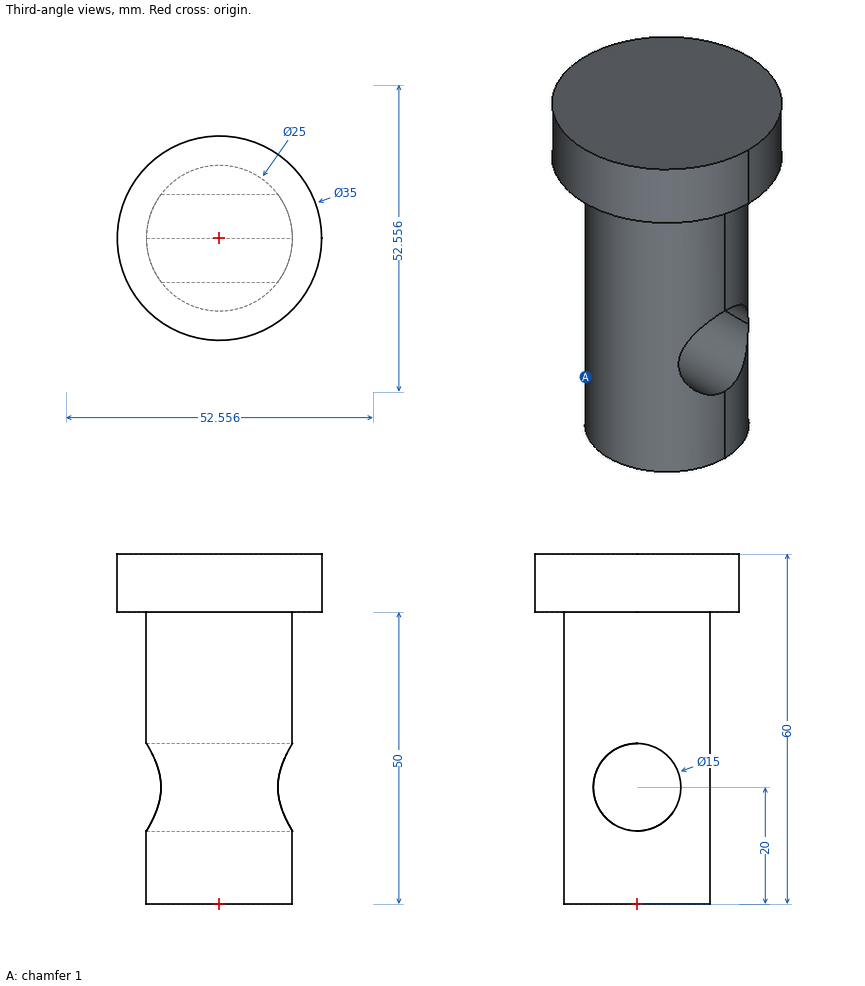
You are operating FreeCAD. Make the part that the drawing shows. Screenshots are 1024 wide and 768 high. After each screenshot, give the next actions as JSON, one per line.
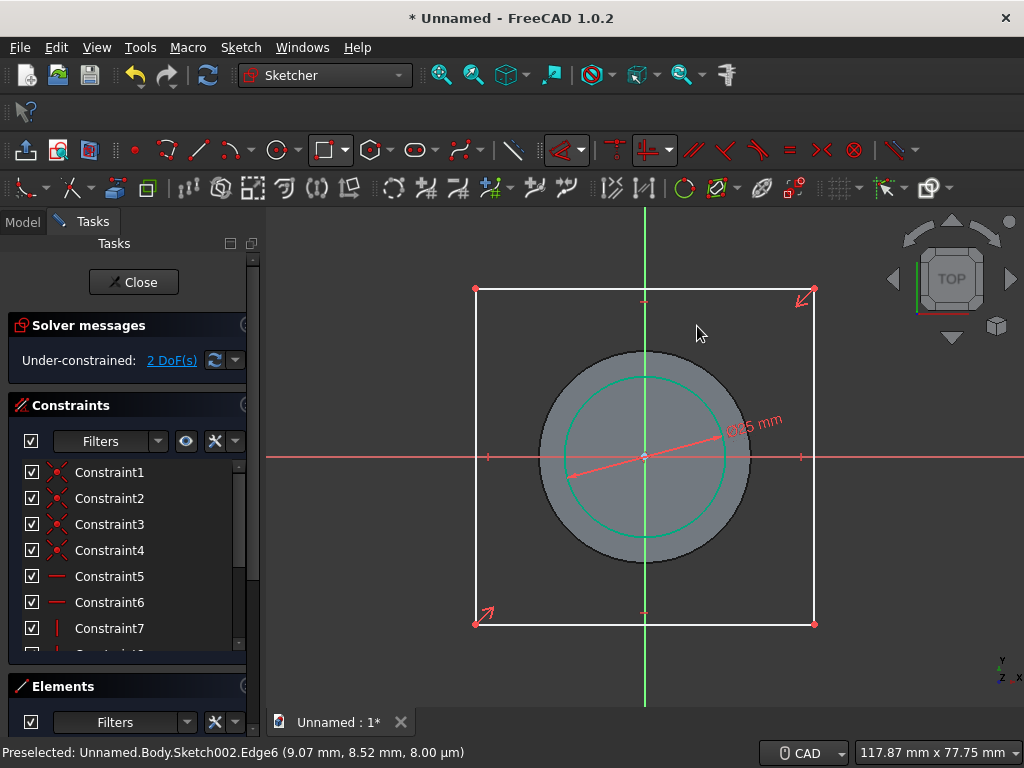
{"action": "left_click", "coordinate": [577, 625]}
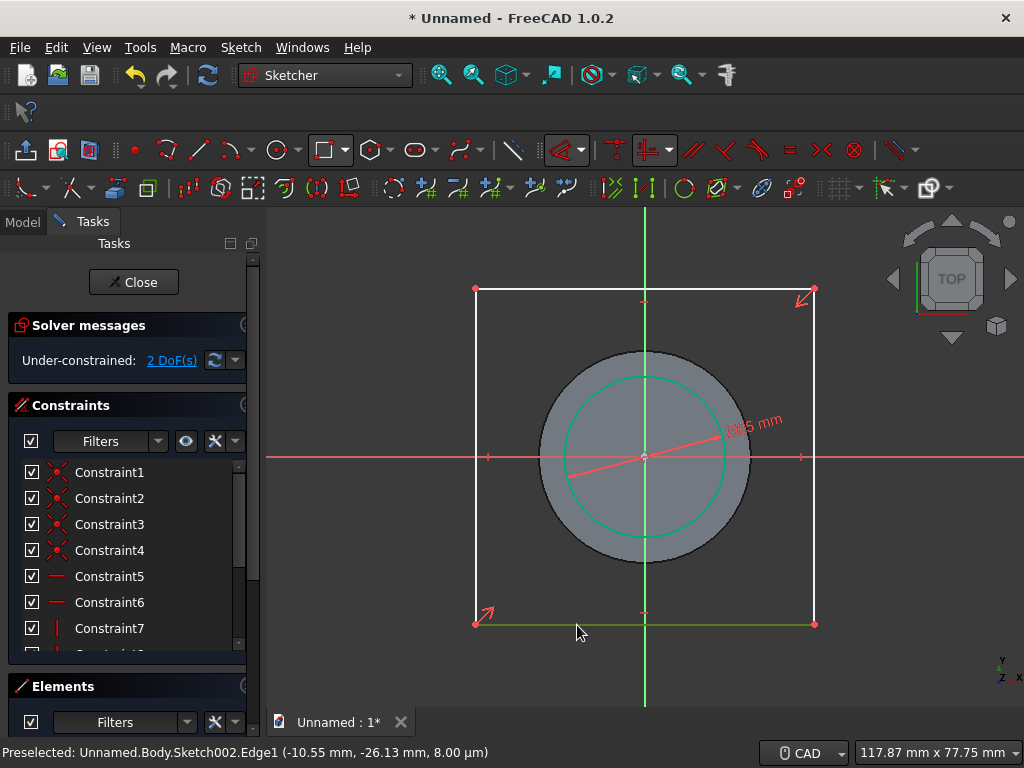
{"action": "left_click", "coordinate": [584, 150]}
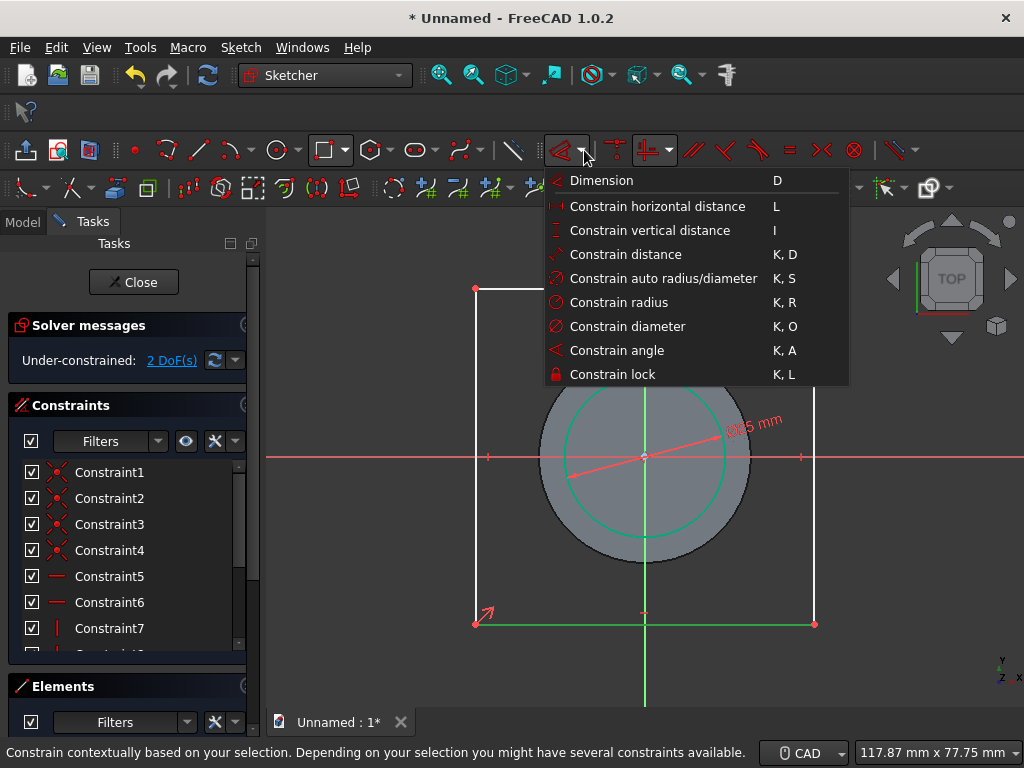
{"action": "left_click", "coordinate": [697, 206]}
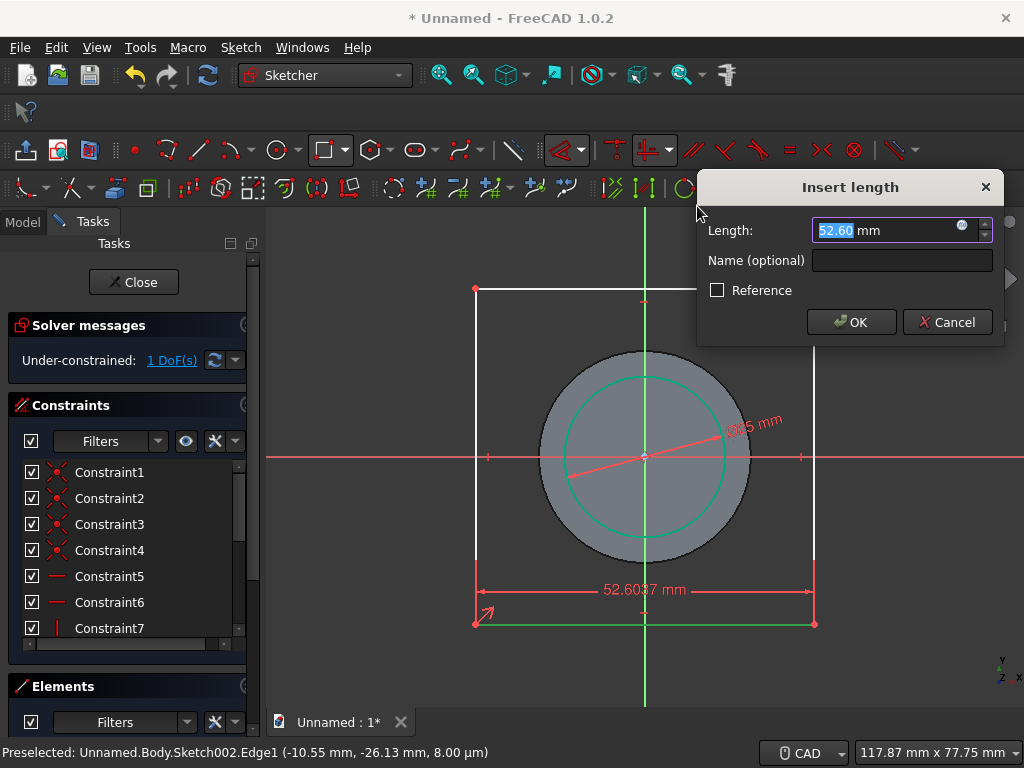
{"action": "type", "text": "52.556"}
{"action": "key", "text": "Return"}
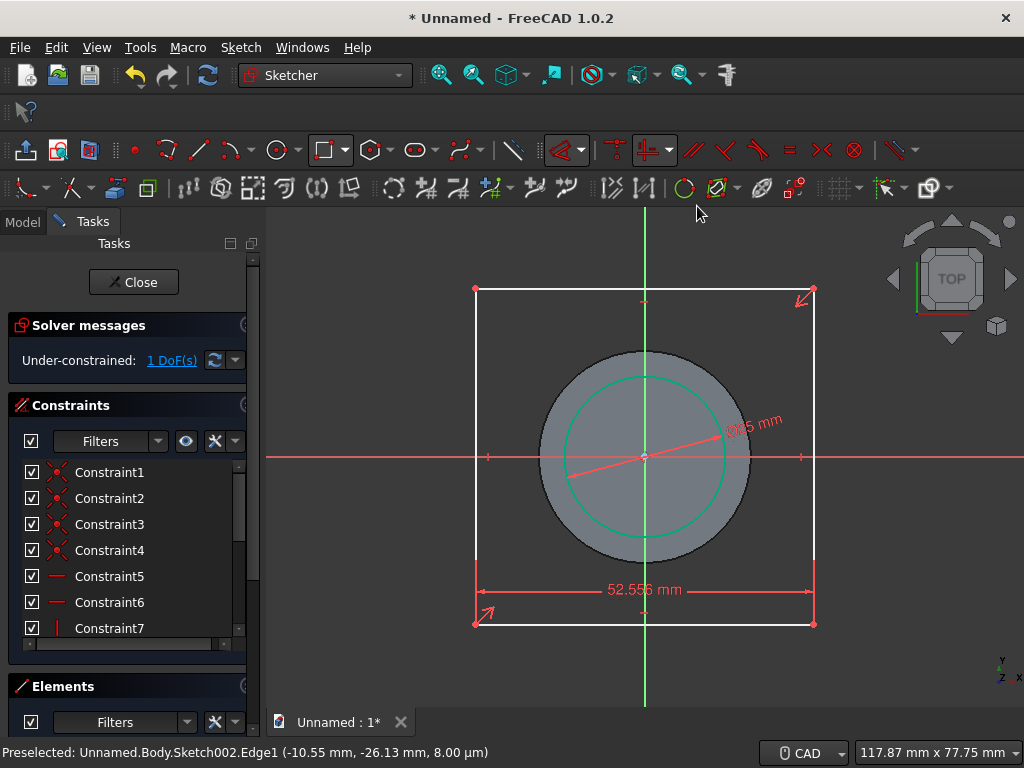
{"action": "left_click", "coordinate": [814, 524]}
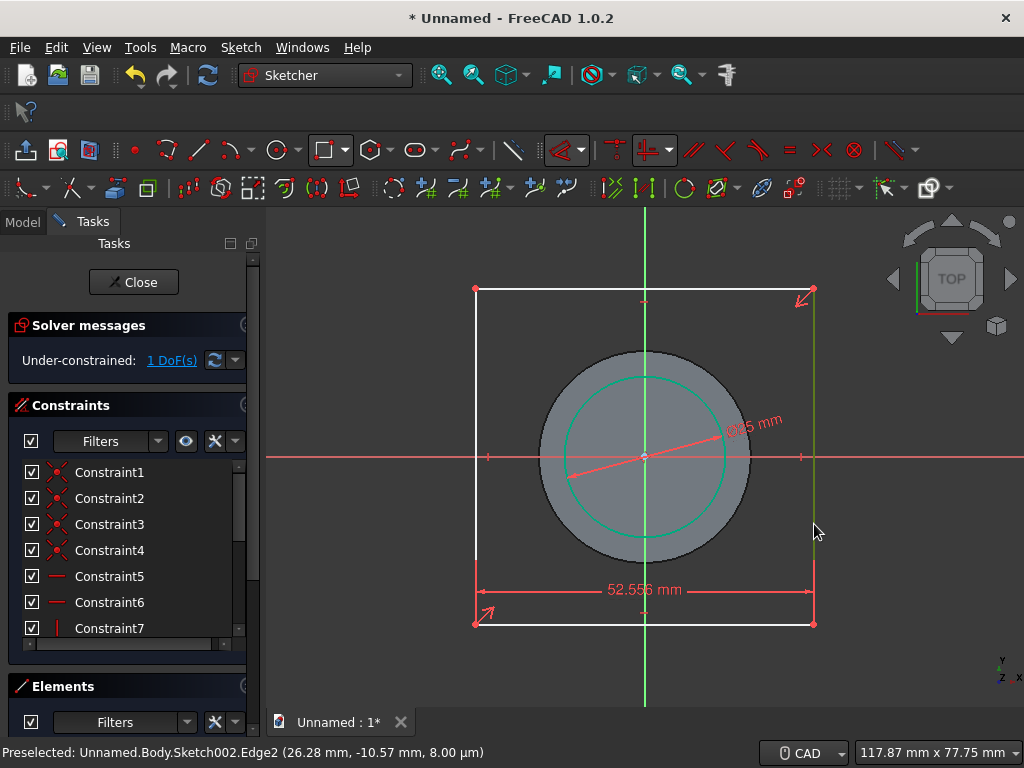
{"action": "key", "text": "i"}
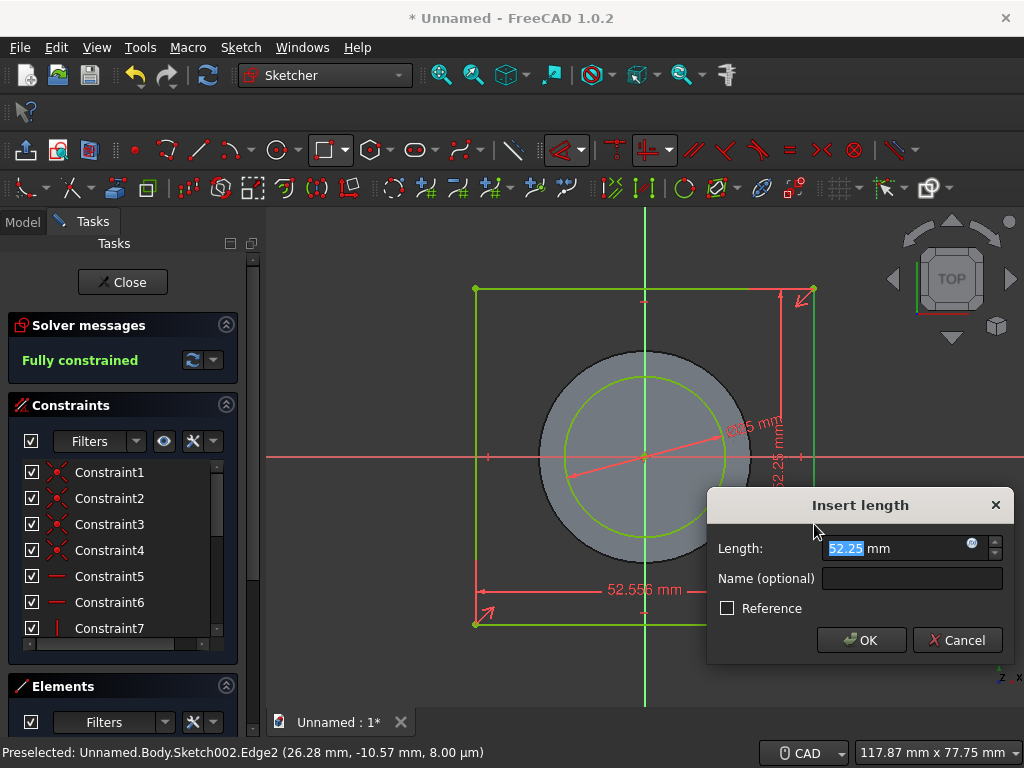
{"action": "type", "text": "52.556"}
{"action": "key", "text": "Return"}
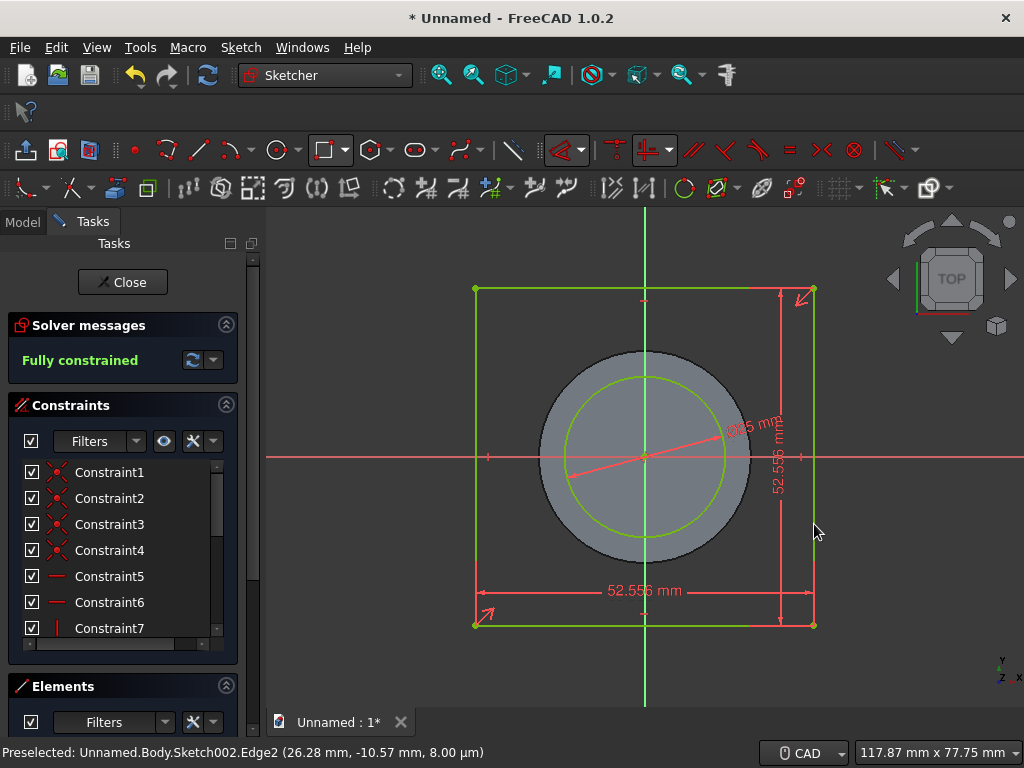
{"action": "left_click", "coordinate": [123, 282]}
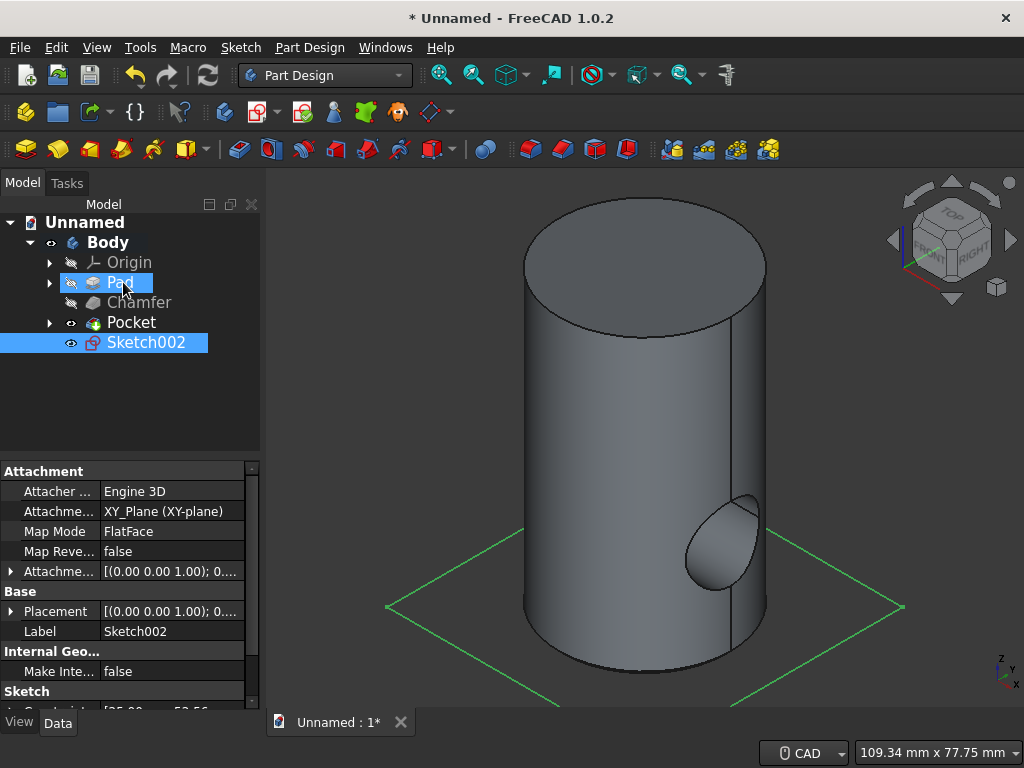
{"action": "left_click", "coordinate": [240, 150]}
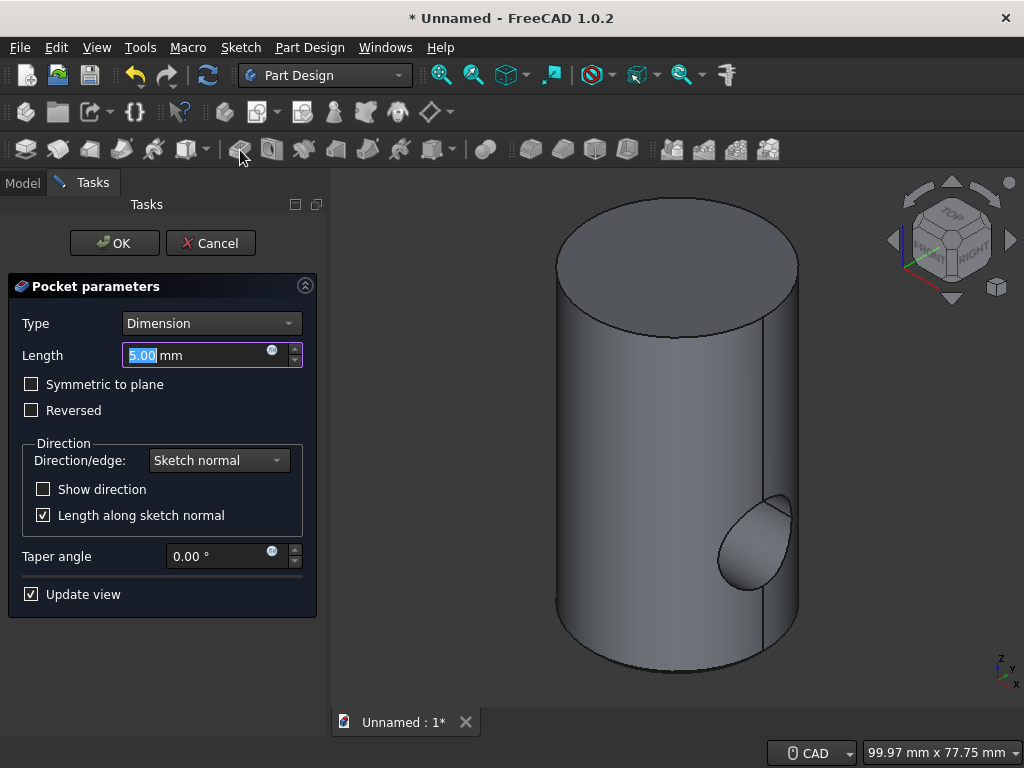
{"action": "type", "text": "50"}
{"action": "key", "text": "Tab"}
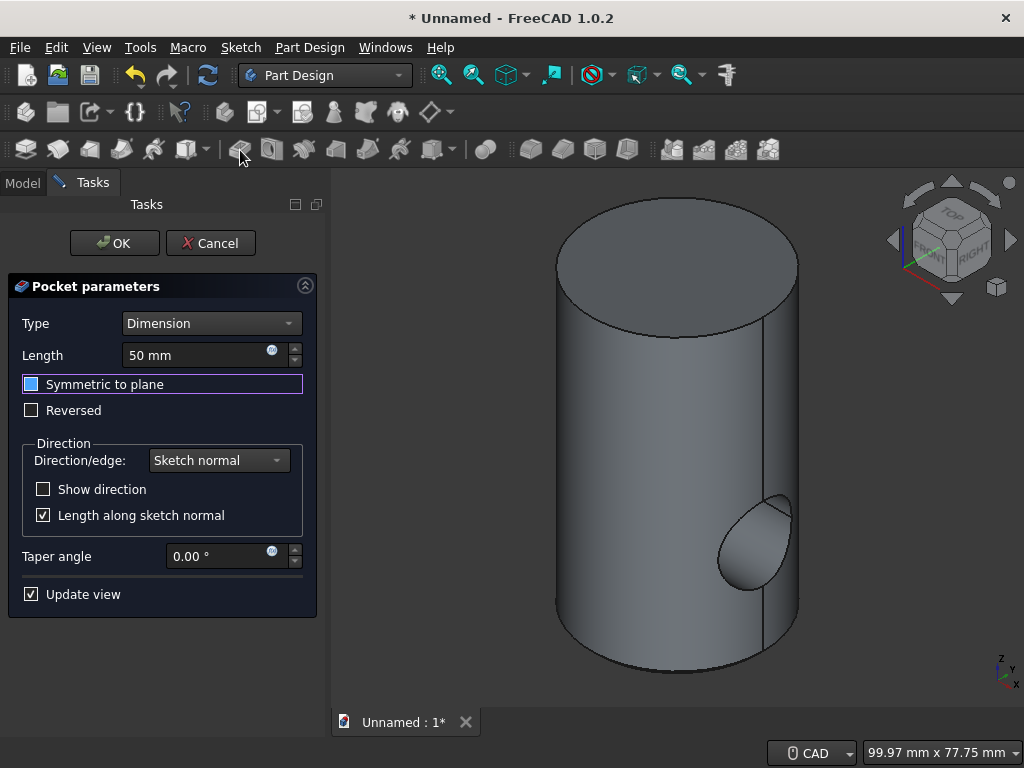
{"action": "left_click", "coordinate": [30, 410]}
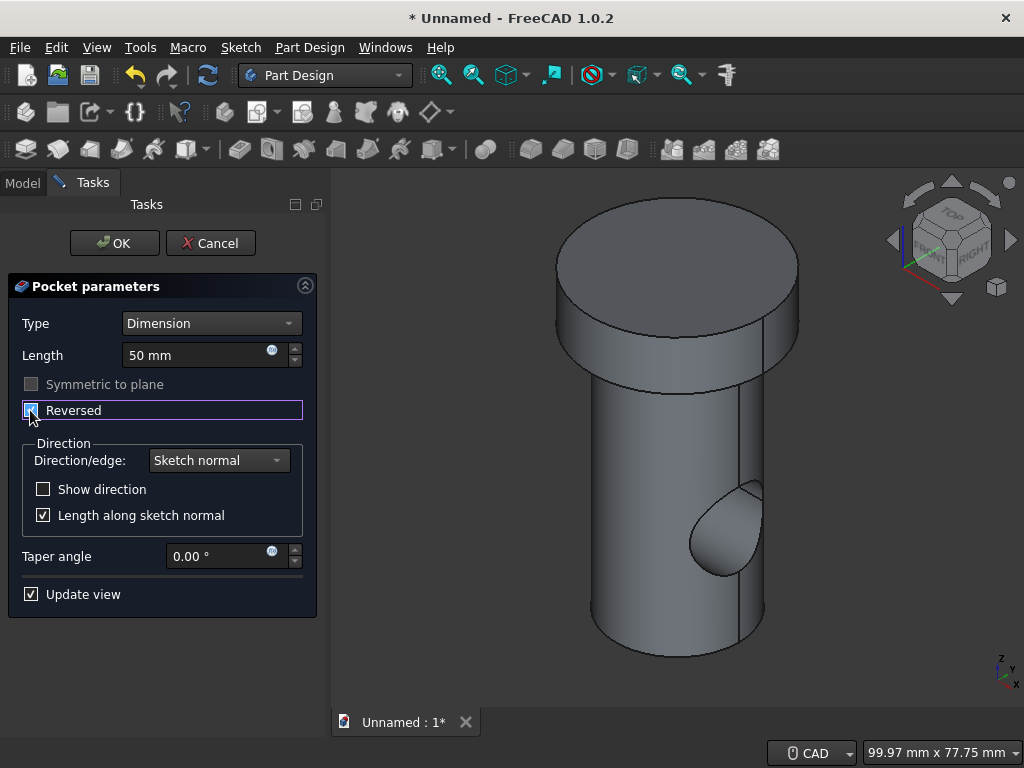
{"action": "left_click", "coordinate": [115, 243]}